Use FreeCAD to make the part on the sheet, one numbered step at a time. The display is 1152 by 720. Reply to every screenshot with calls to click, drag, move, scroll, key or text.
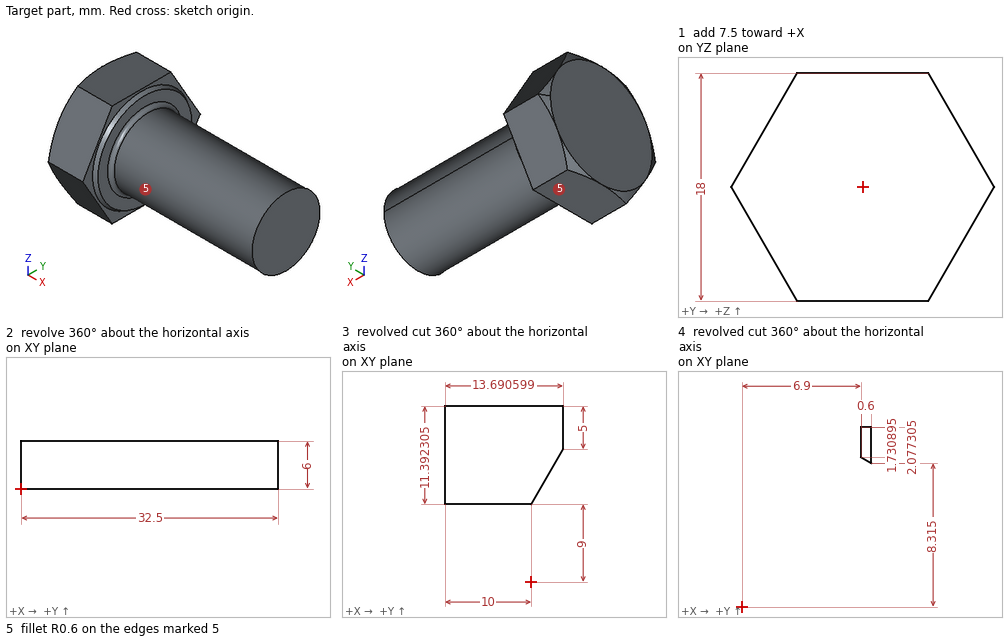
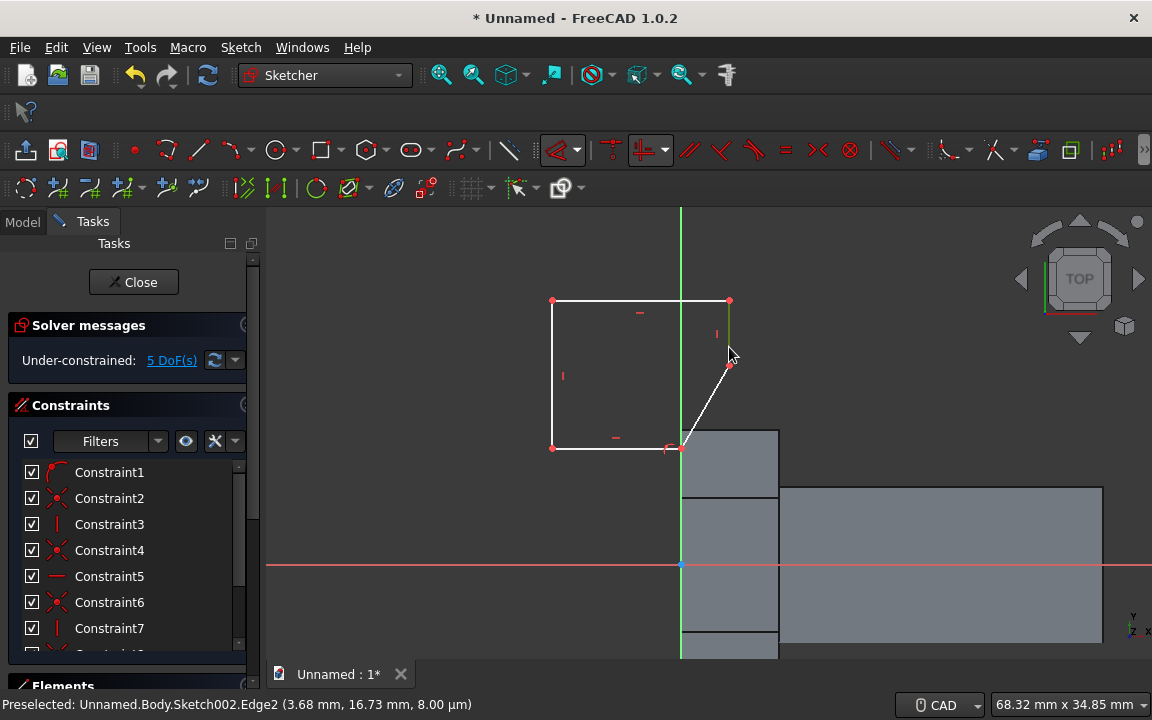
key(i)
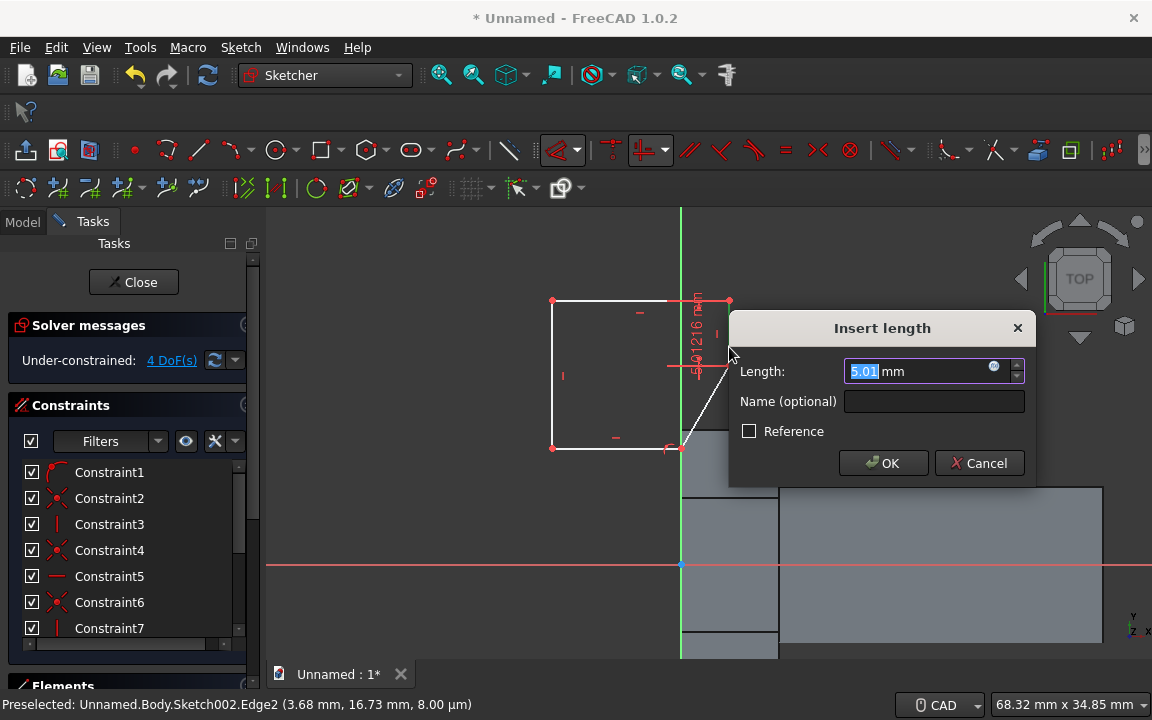
text(5)
key(Return)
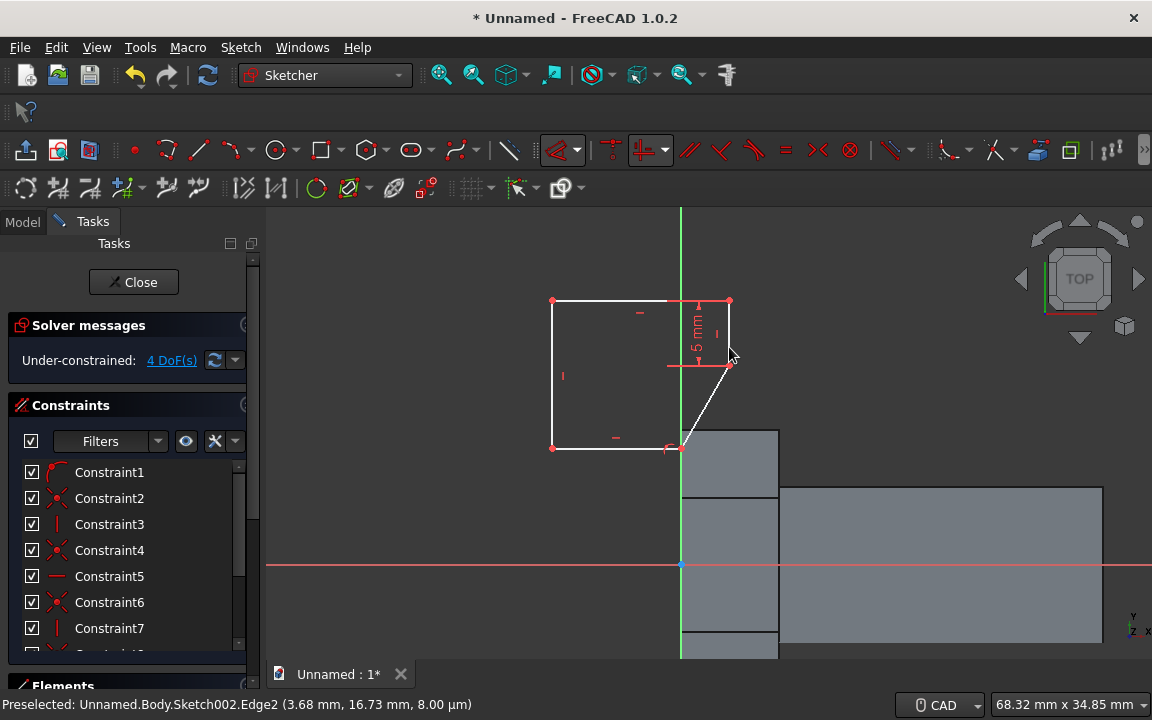
click(591, 449)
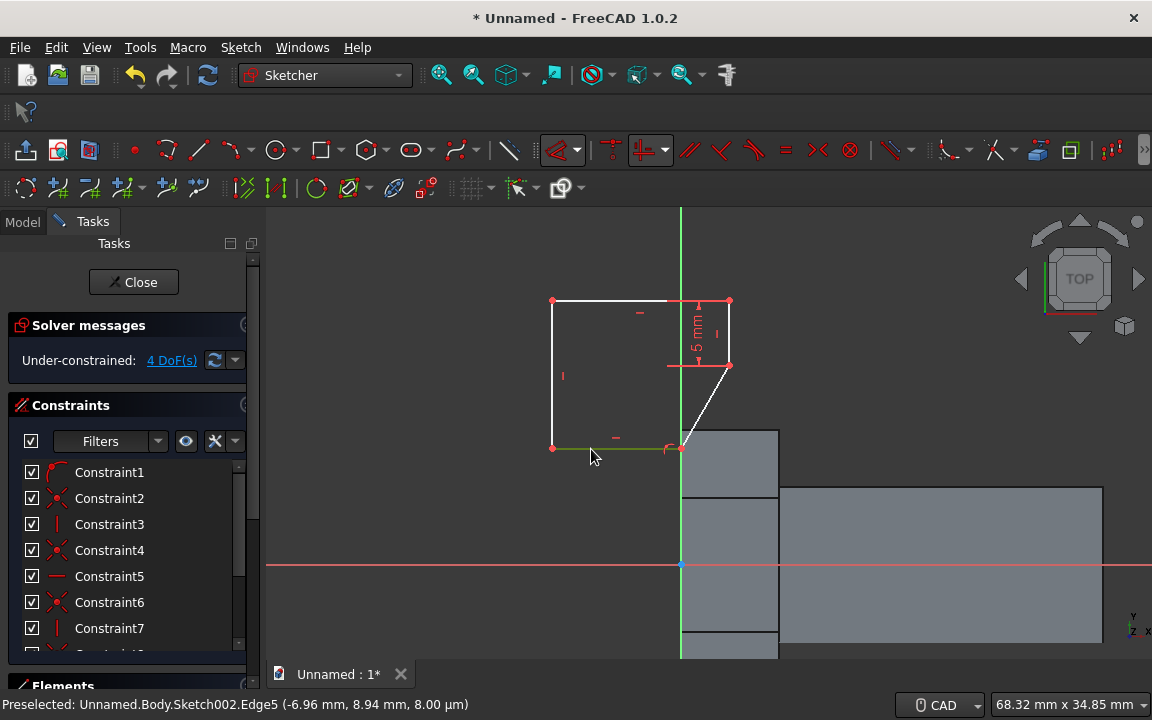
click(580, 150)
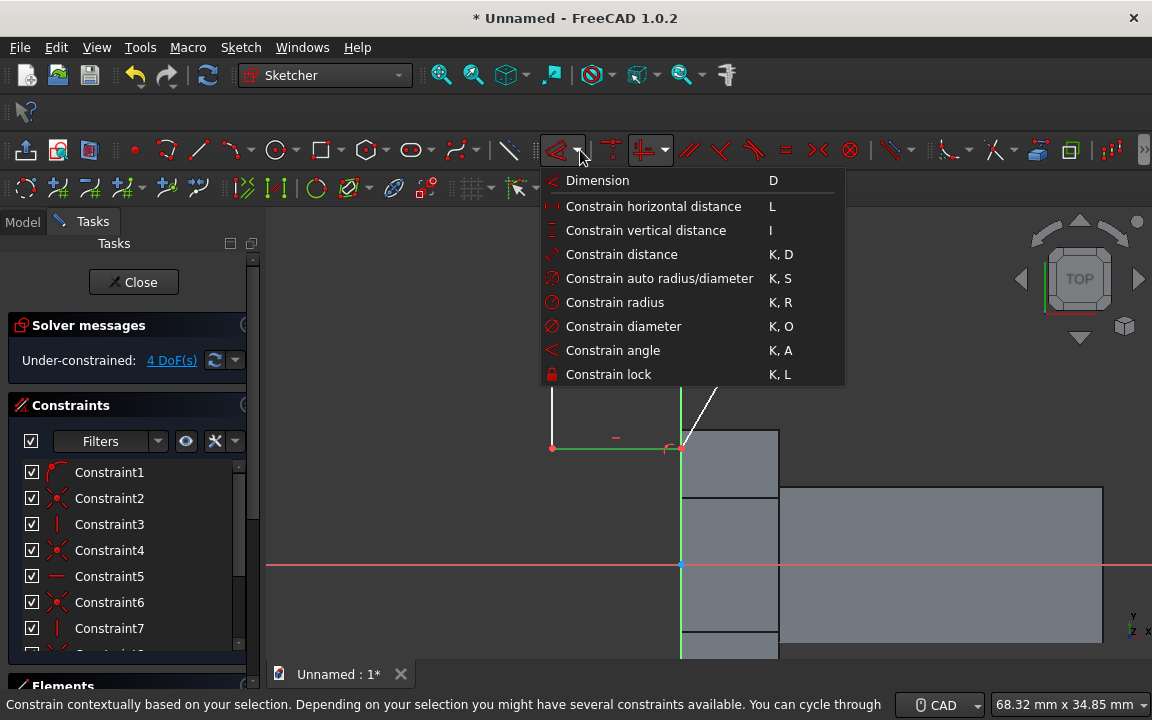
click(693, 206)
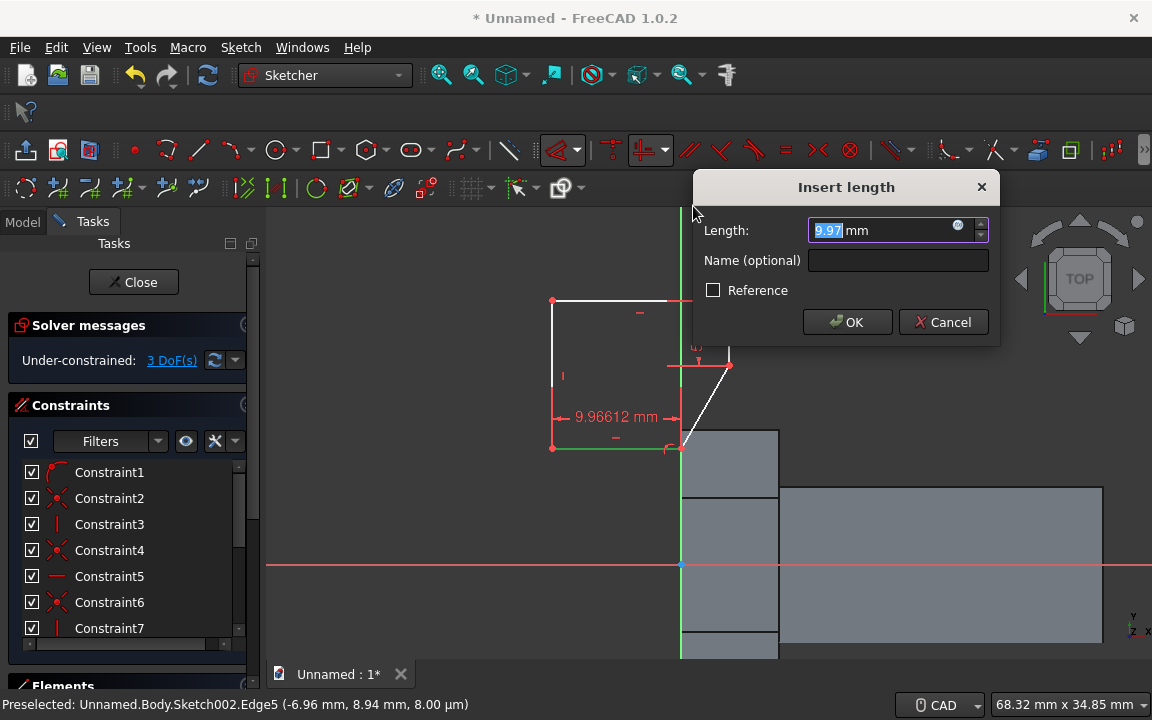
text(10)
key(Return)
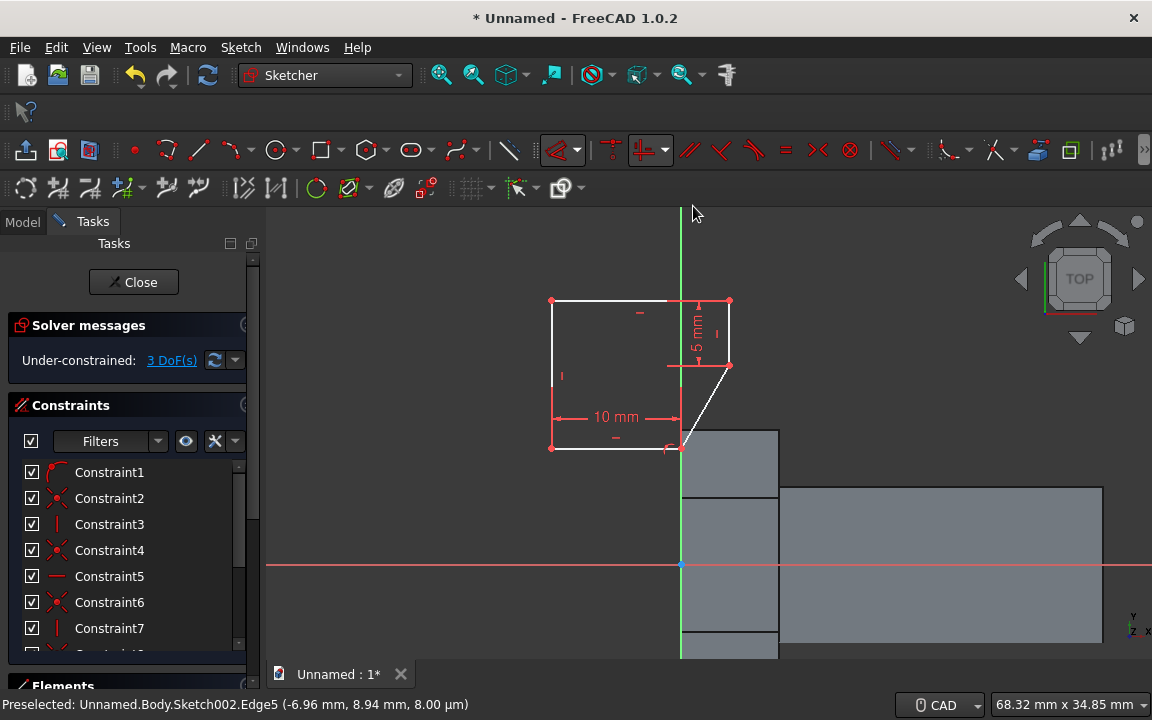
click(681, 449)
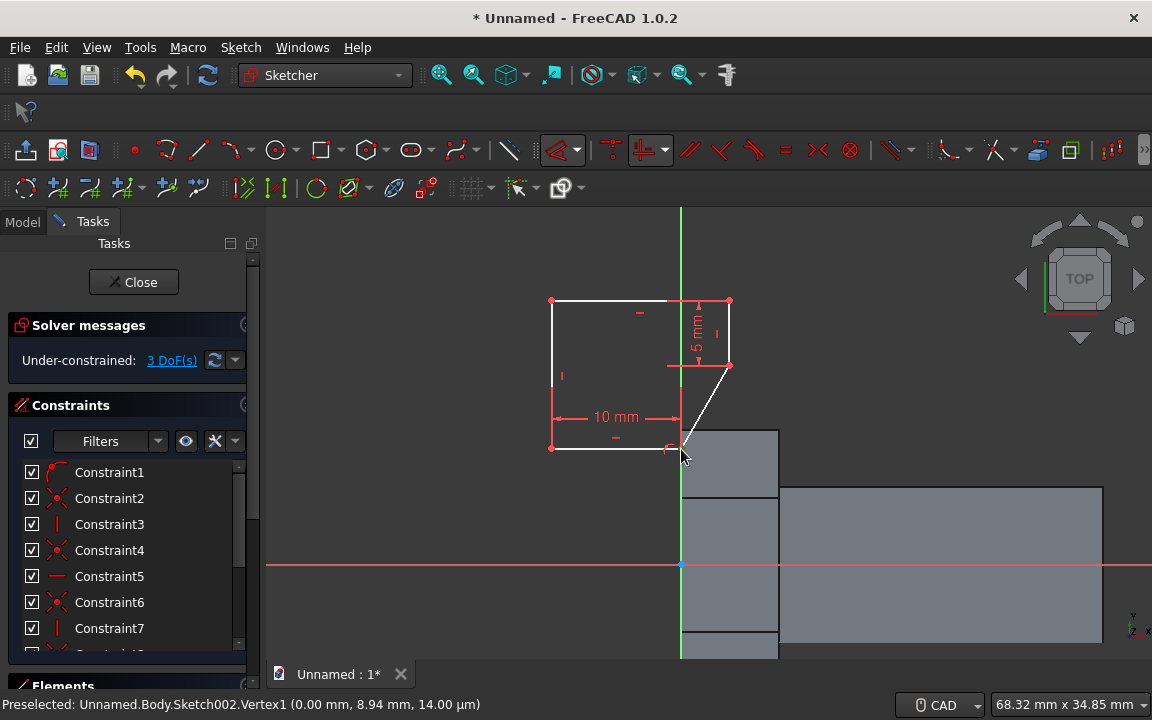
click(580, 150)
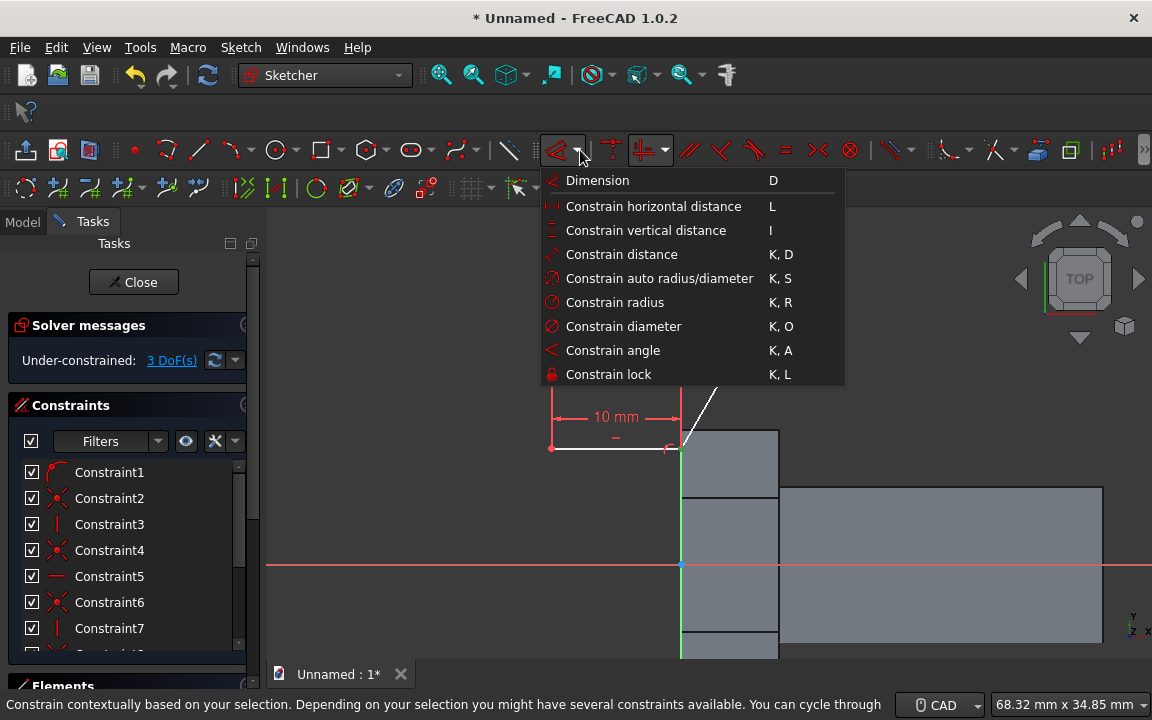
click(693, 230)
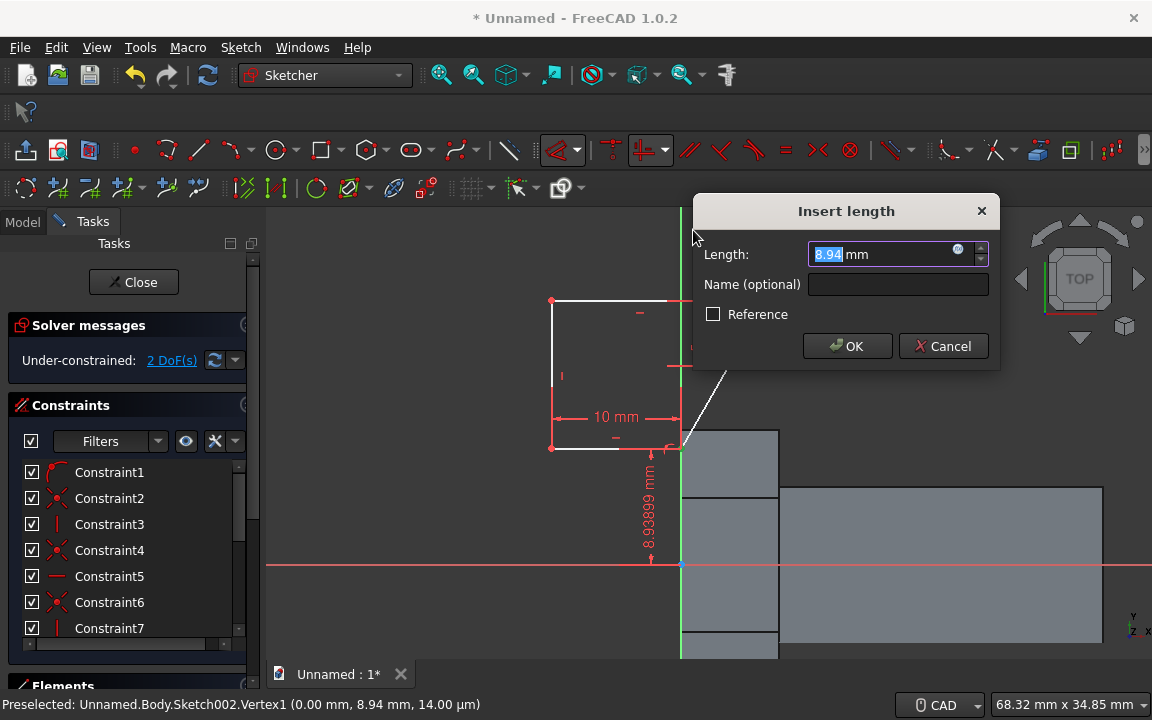
text(9)
key(Return)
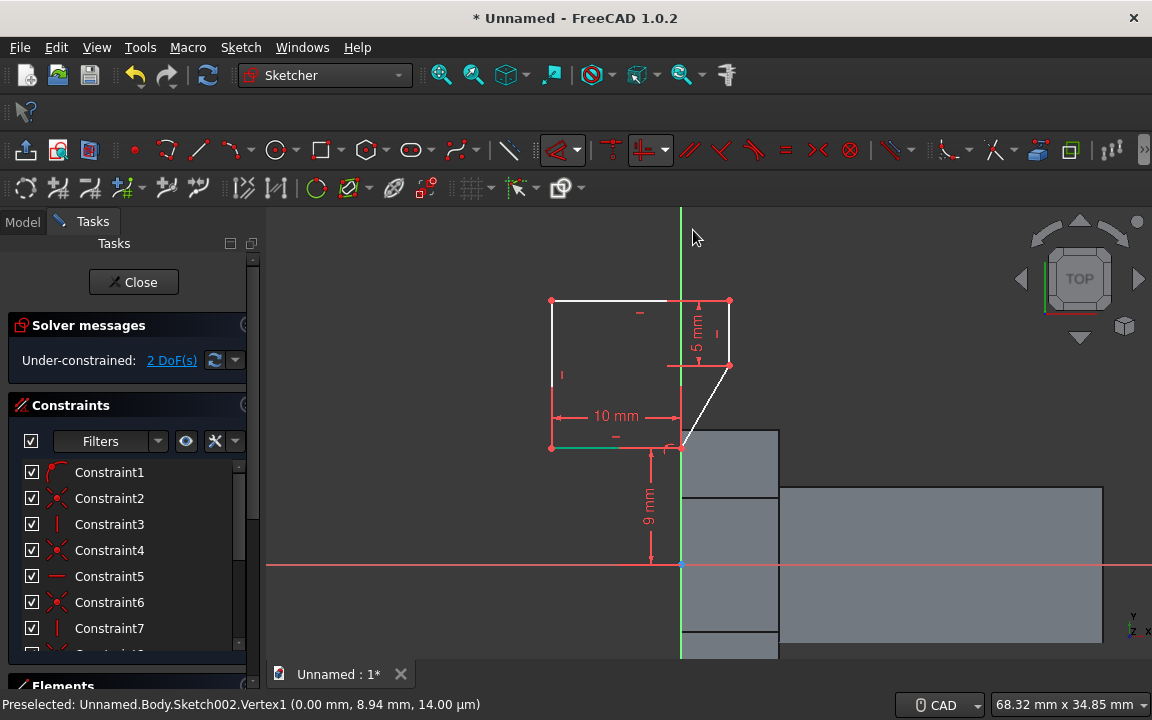
click(605, 301)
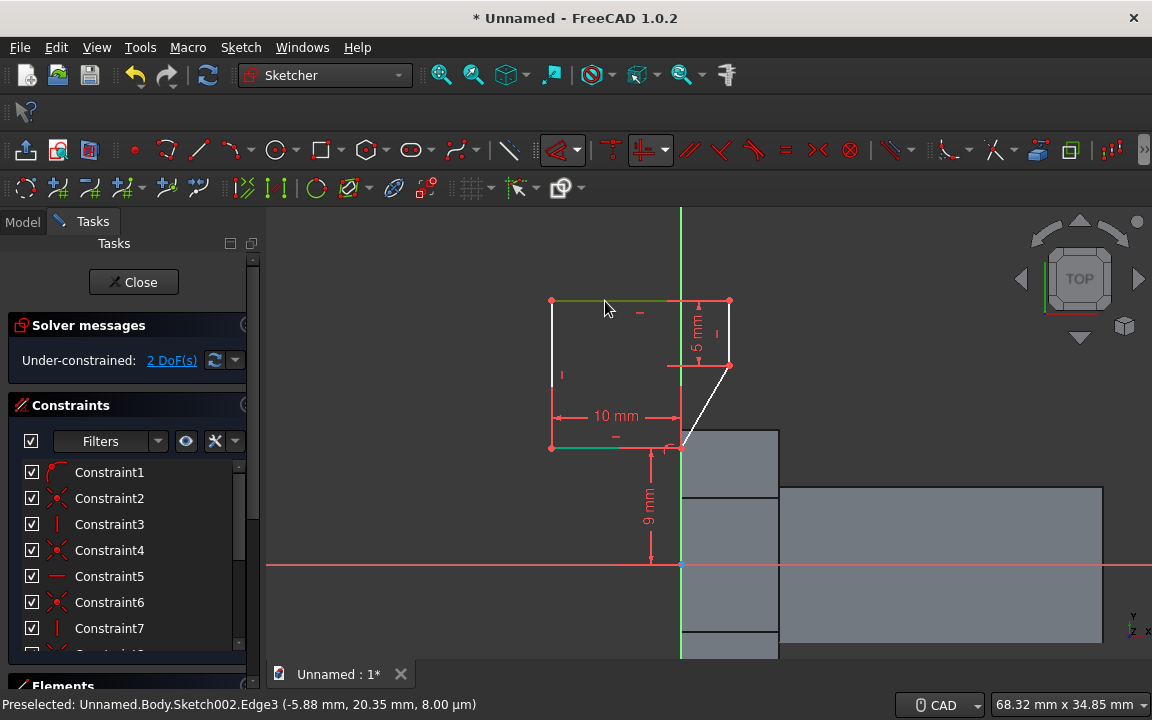
key(l)